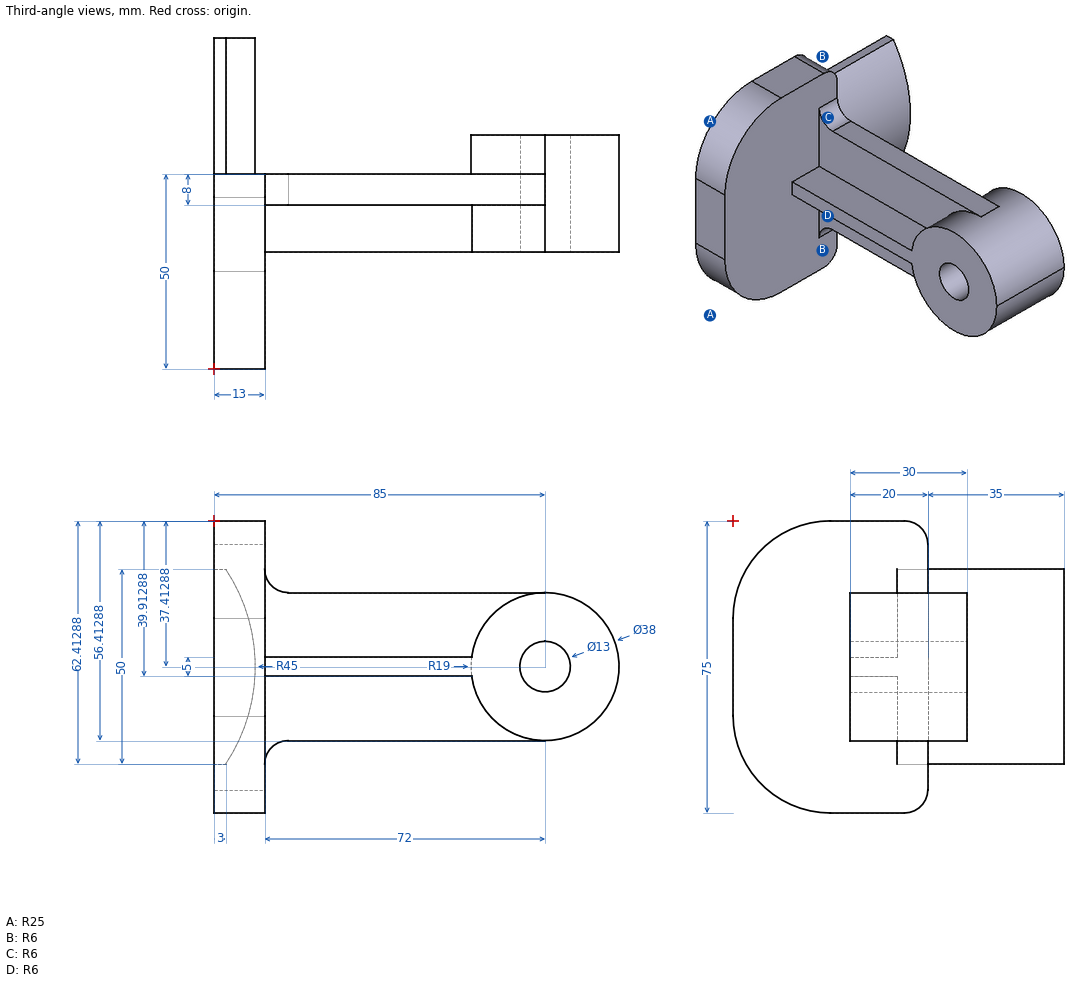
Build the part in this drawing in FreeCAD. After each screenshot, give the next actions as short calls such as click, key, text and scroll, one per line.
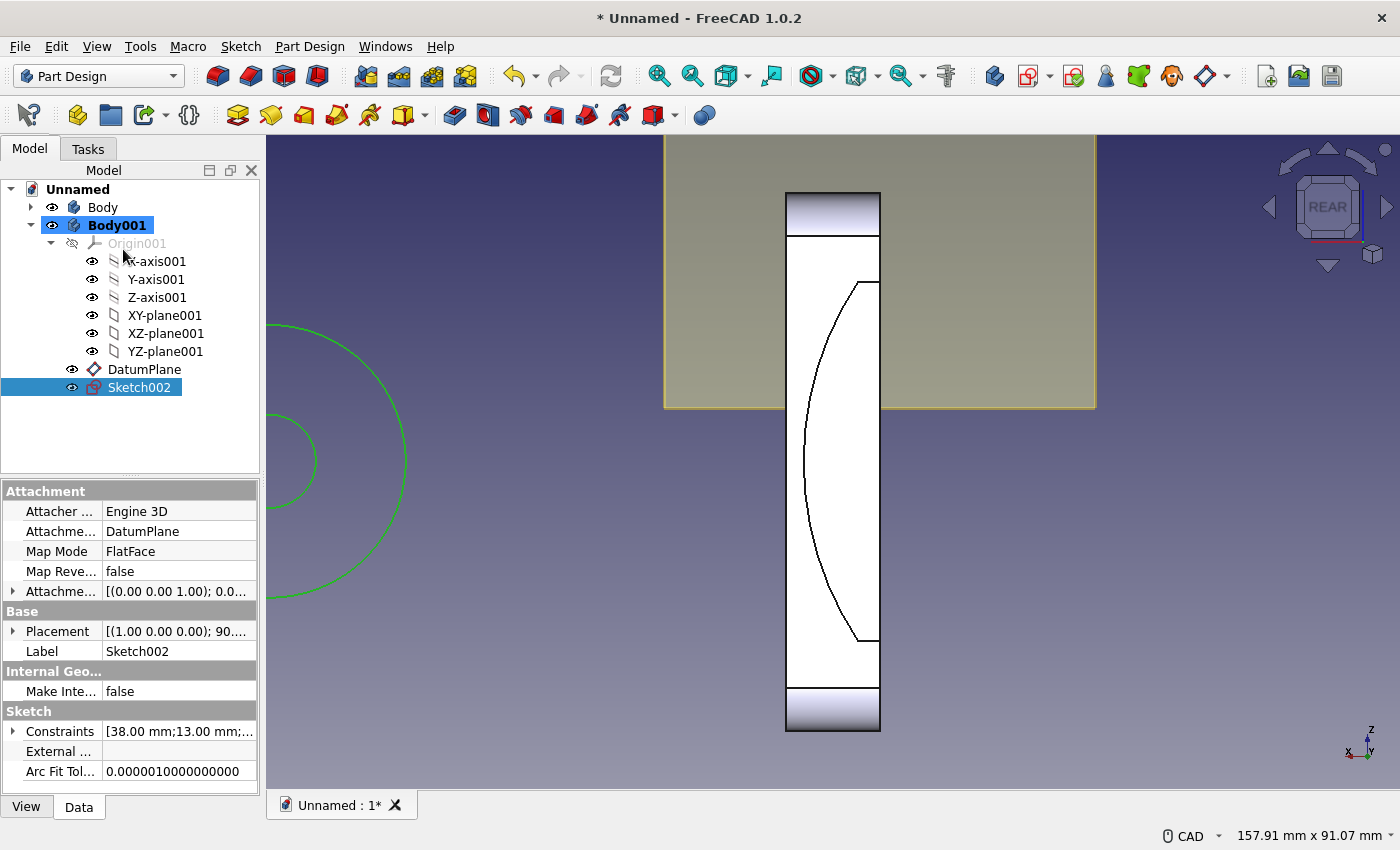
click(238, 116)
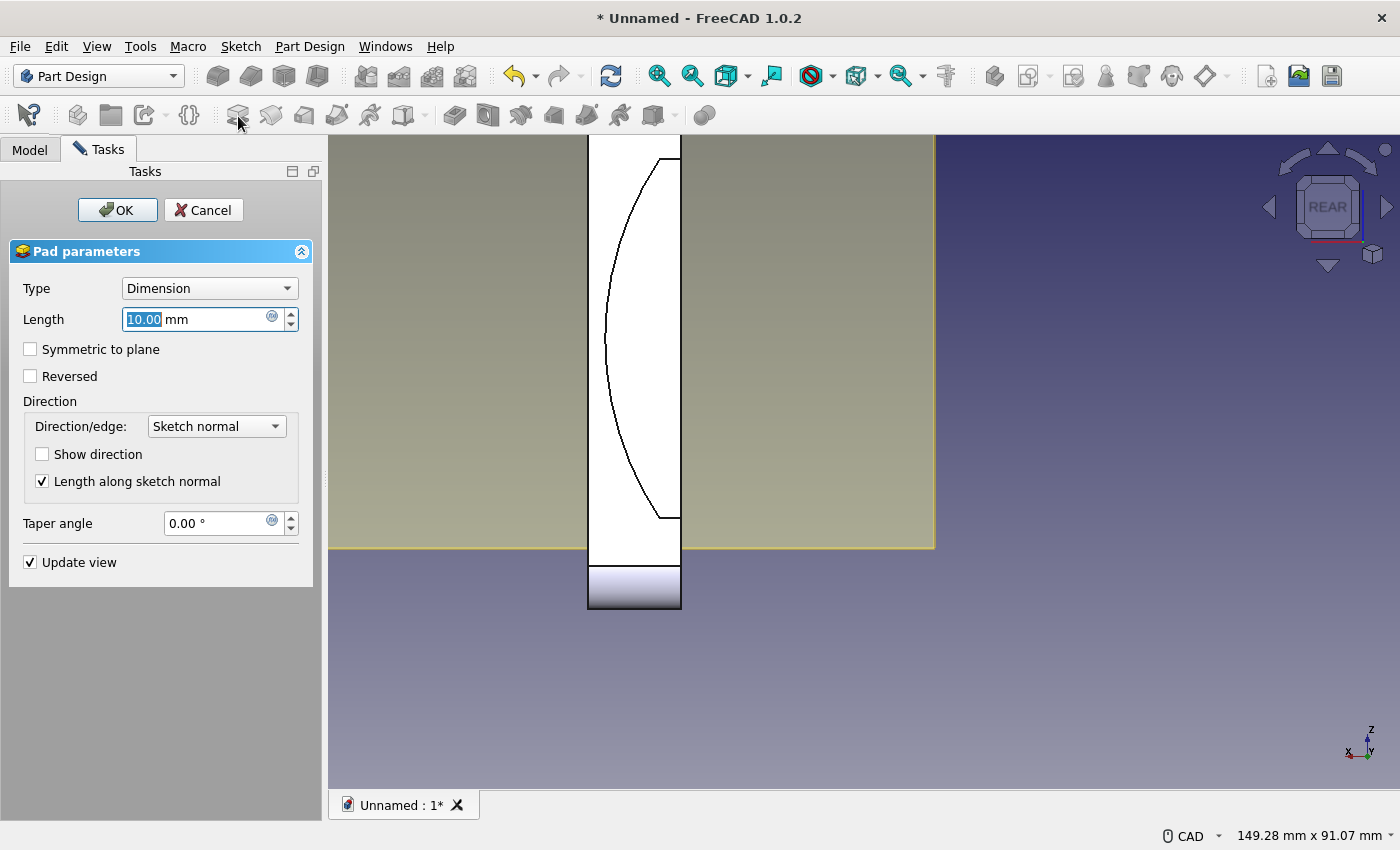
text(30)
key(Tab)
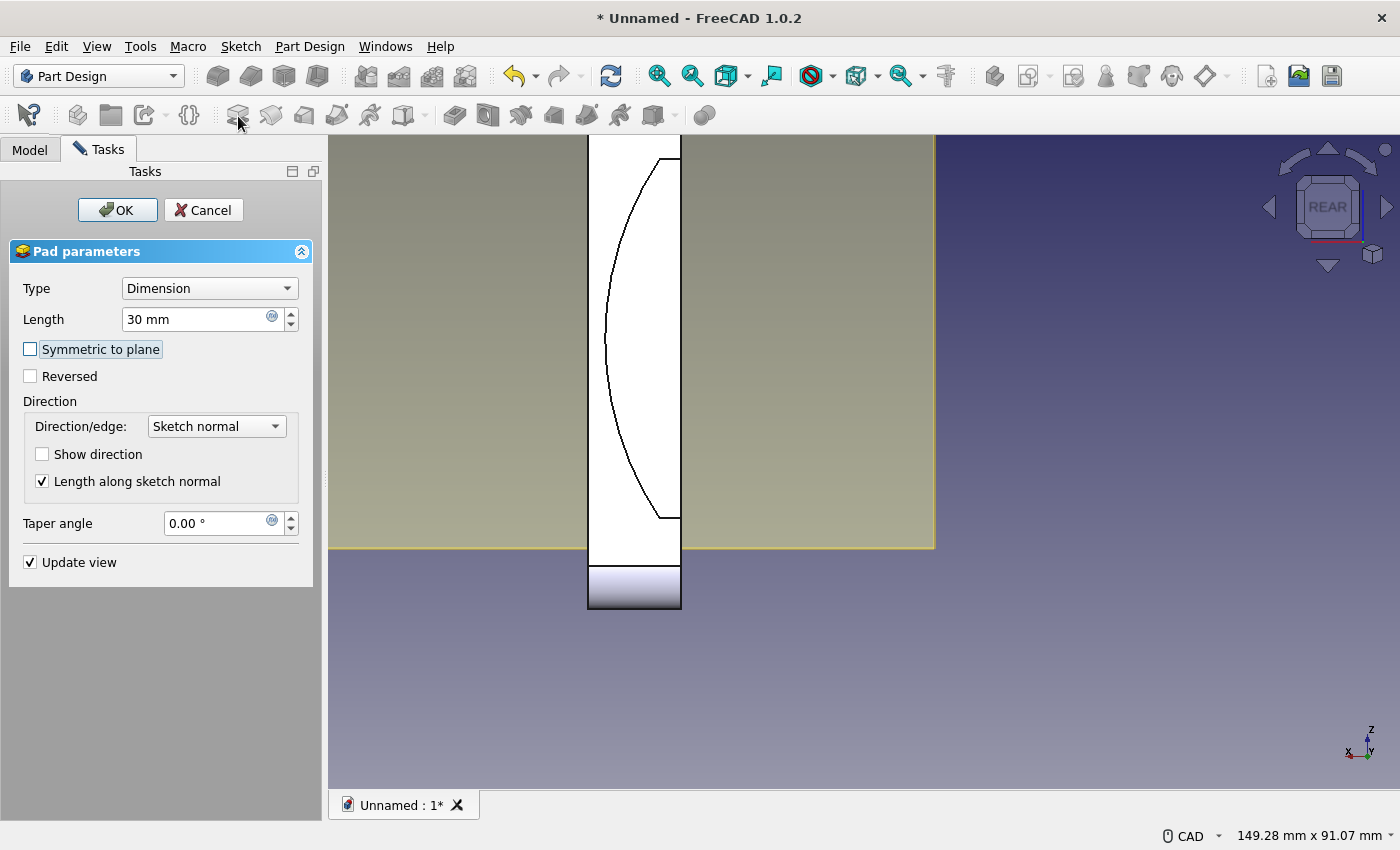
click(31, 376)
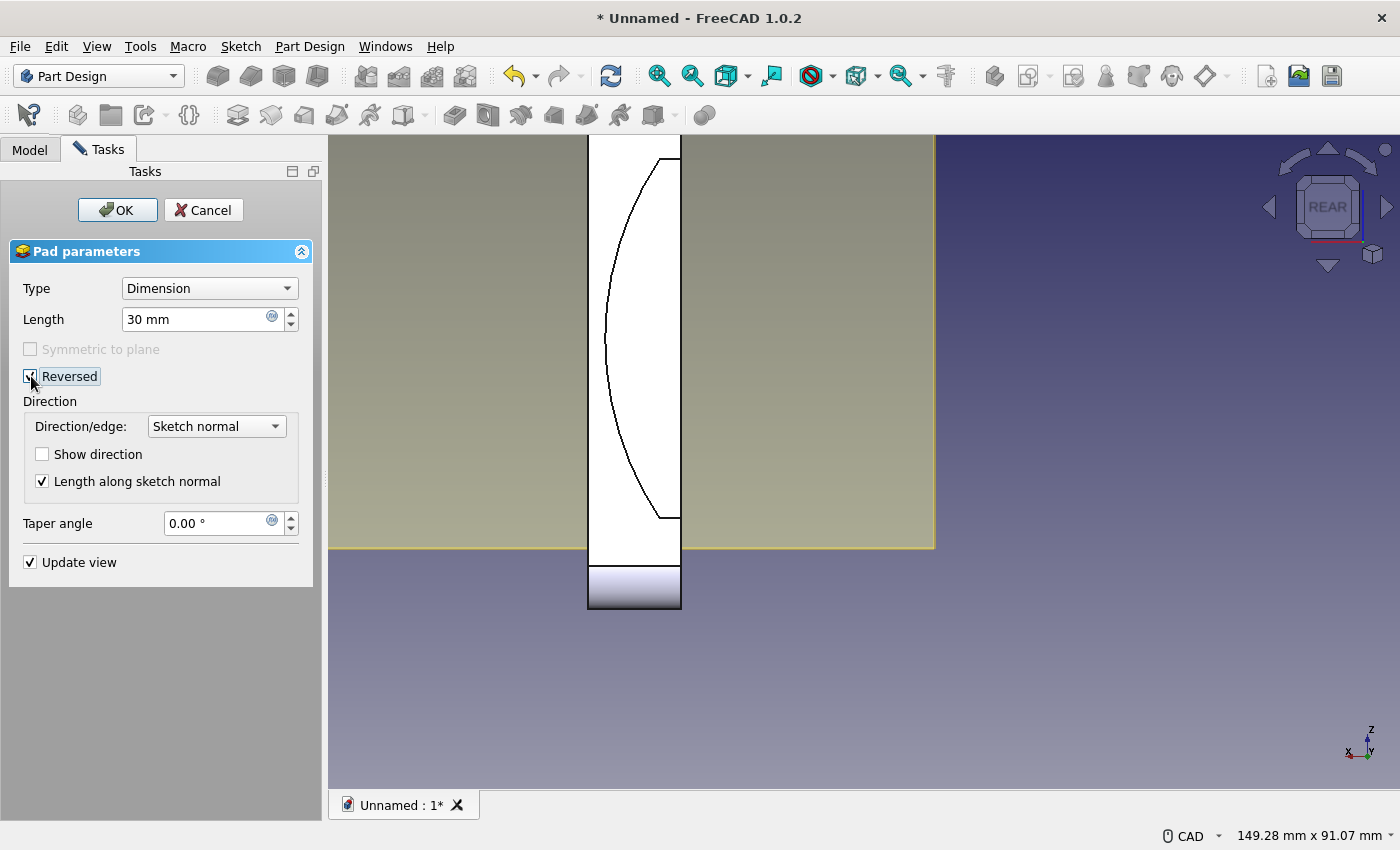
click(118, 210)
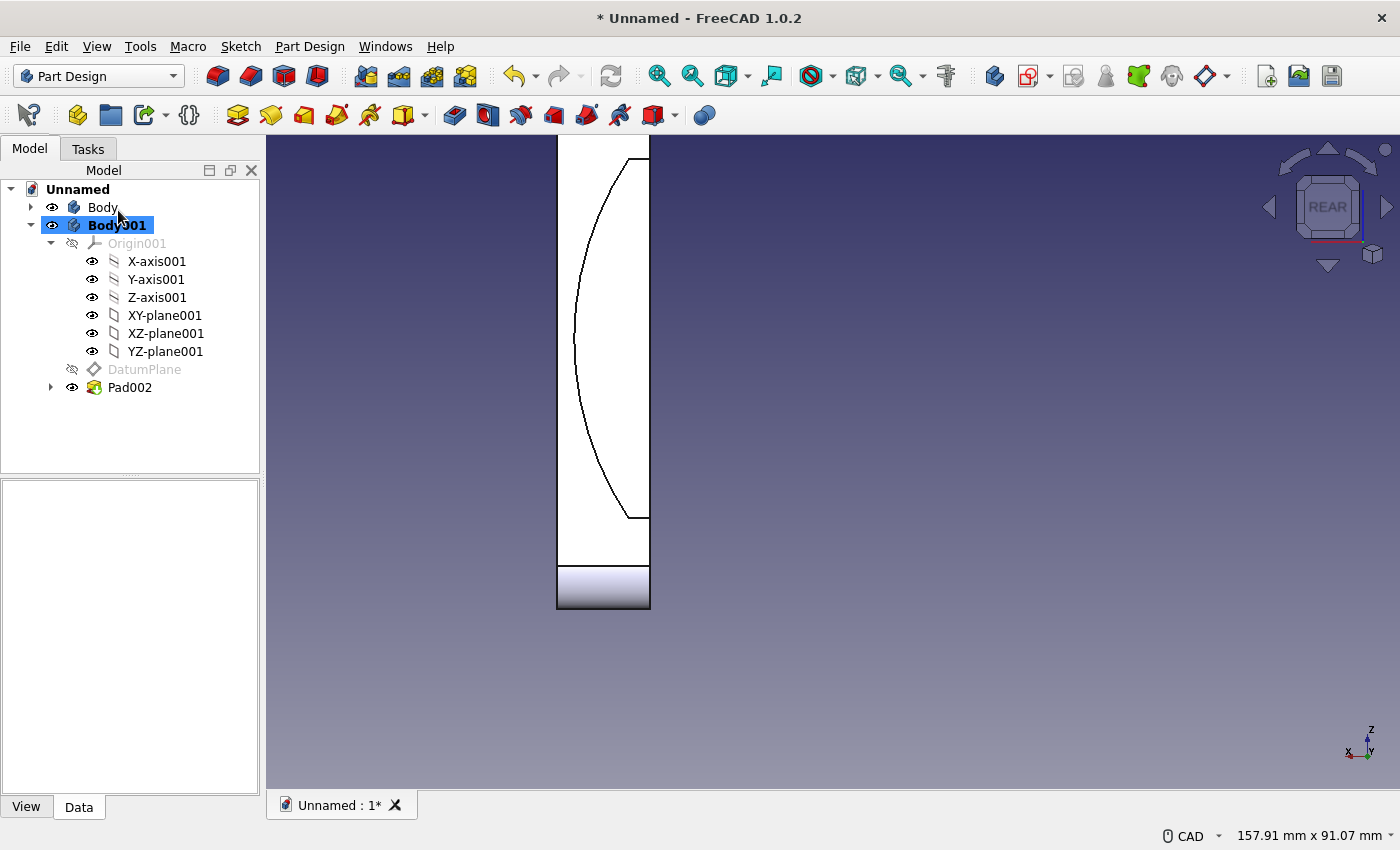
click(660, 76)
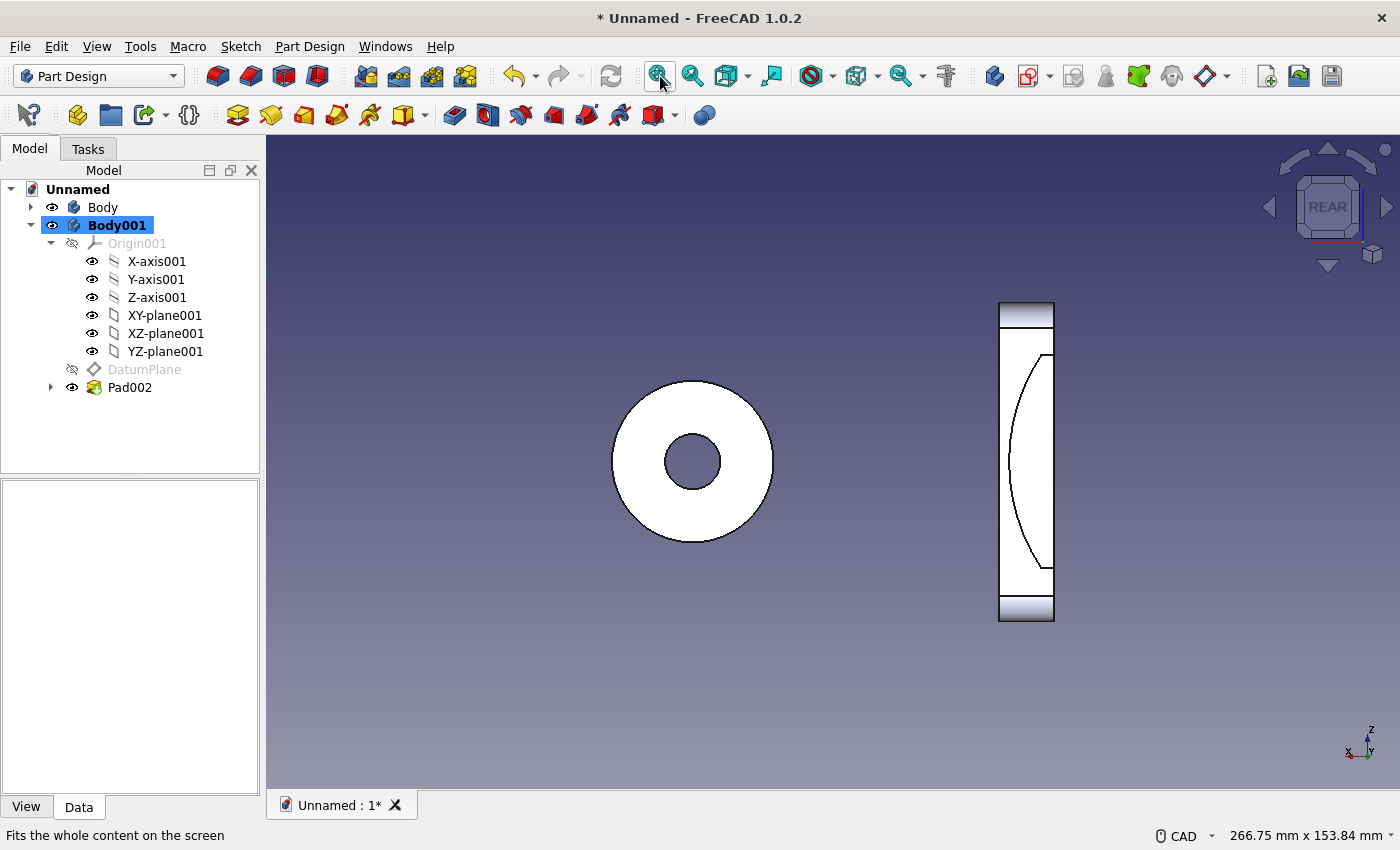
double_click(97, 207)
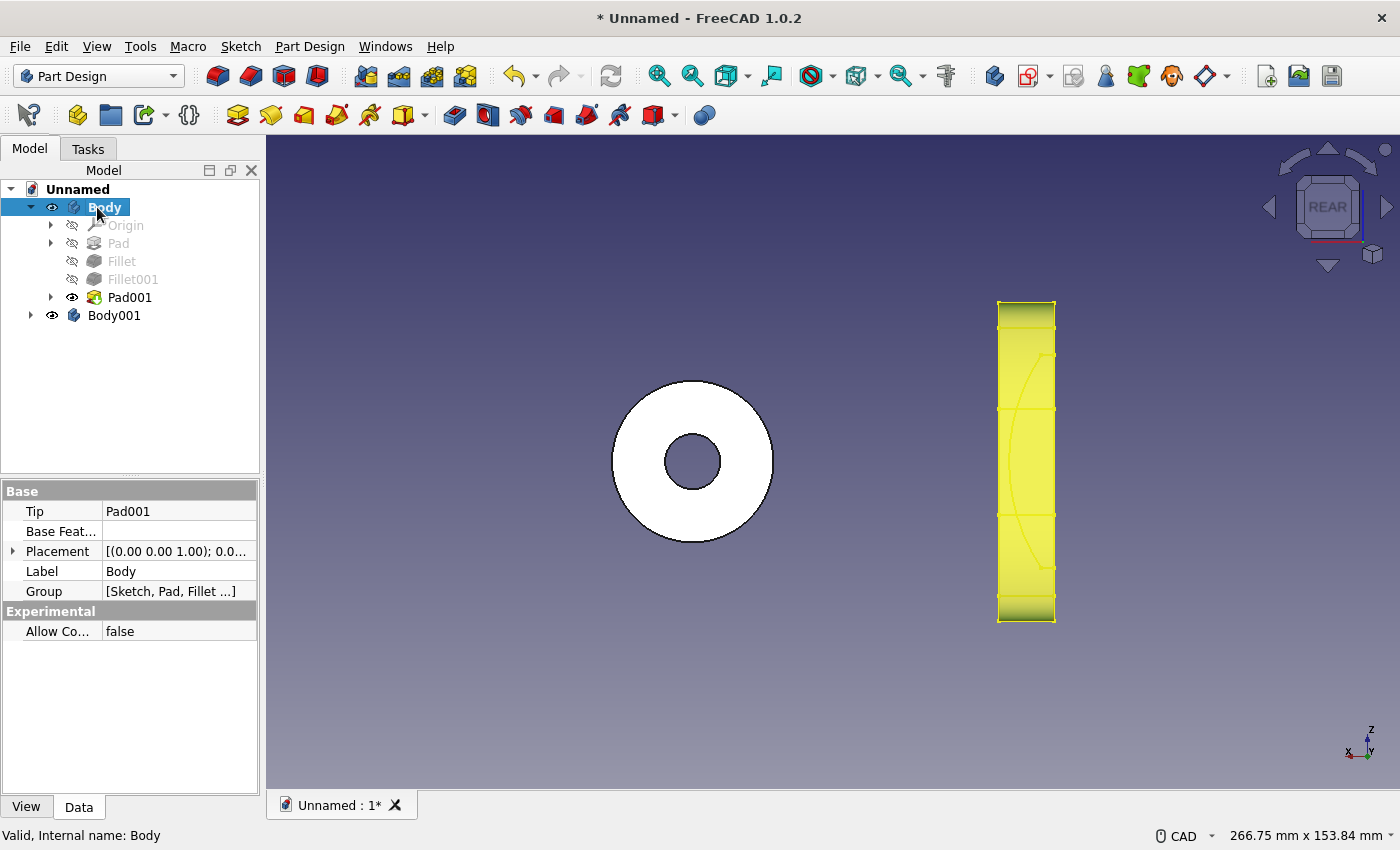
click(97, 207)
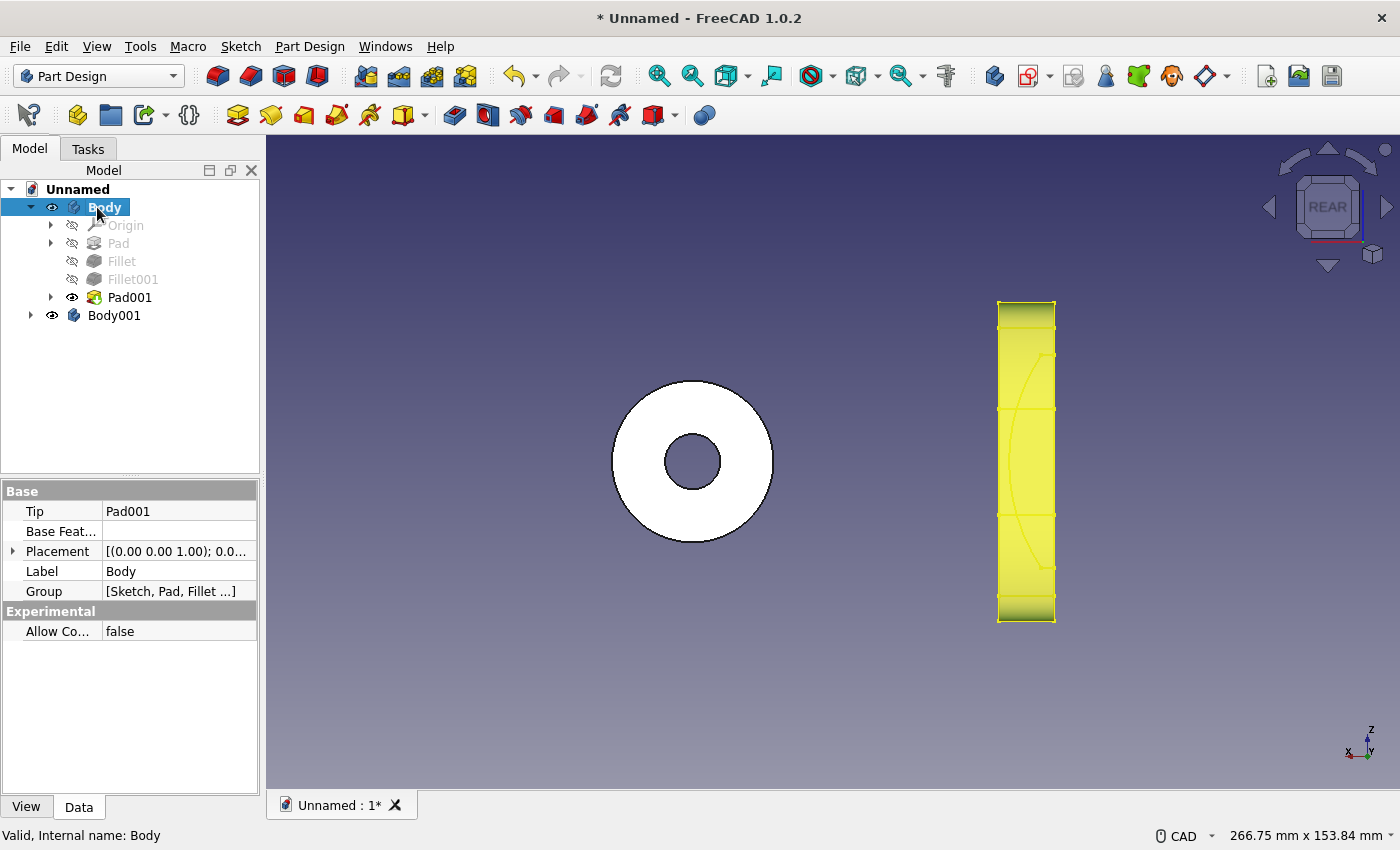
click(148, 631)